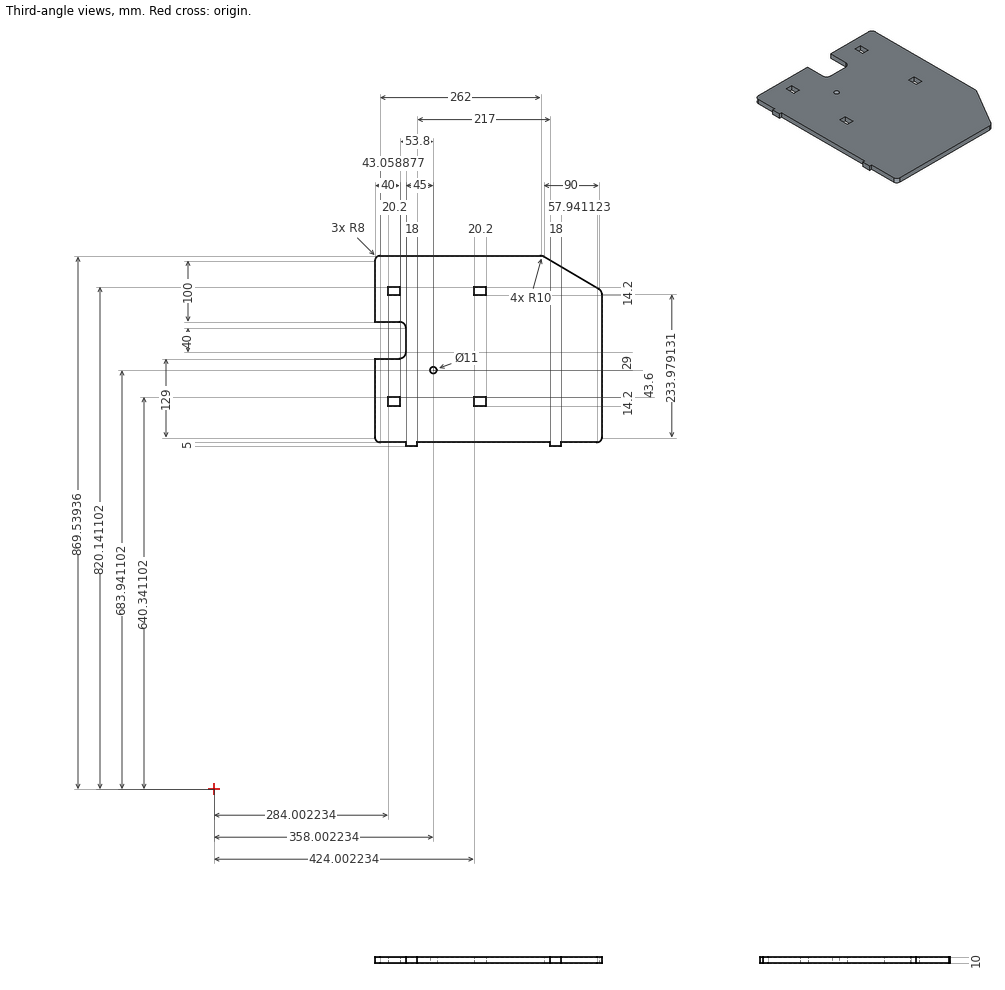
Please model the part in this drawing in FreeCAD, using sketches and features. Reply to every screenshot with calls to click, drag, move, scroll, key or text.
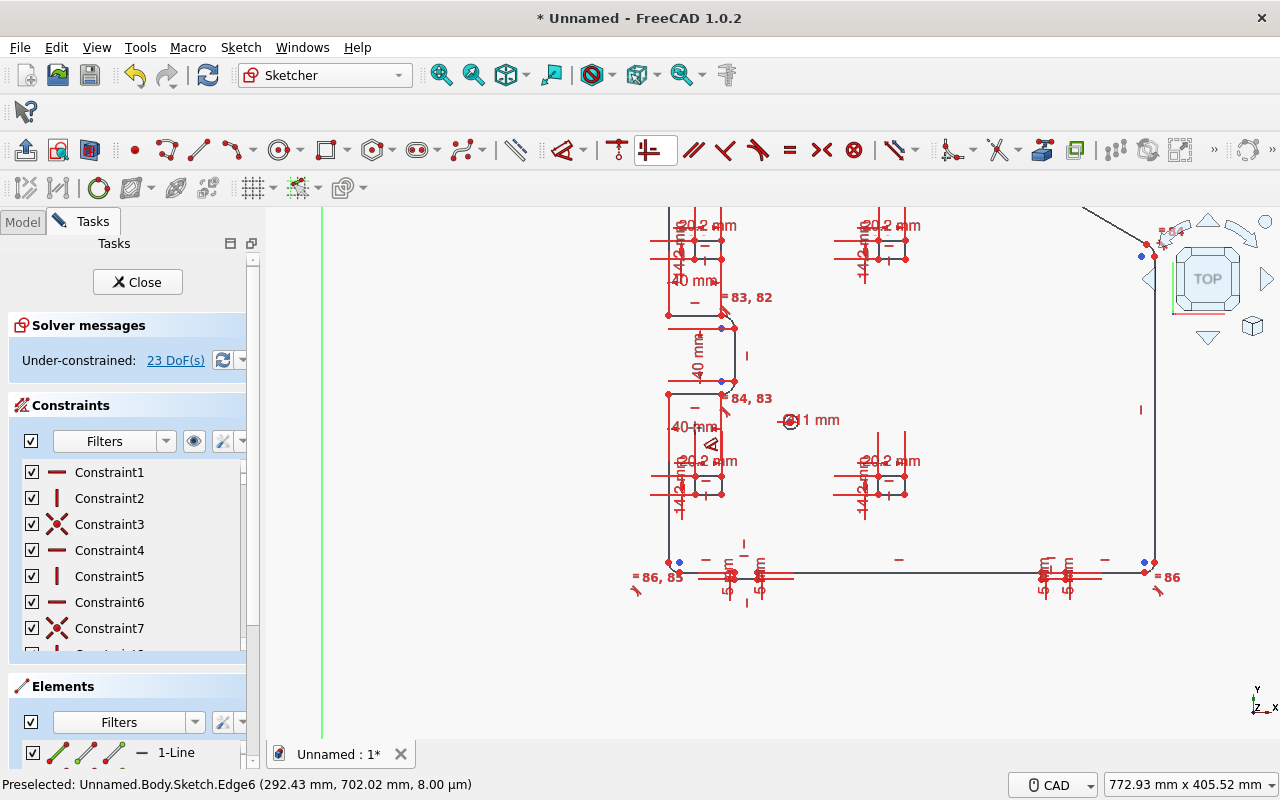
scroll(744, 579, up, 3)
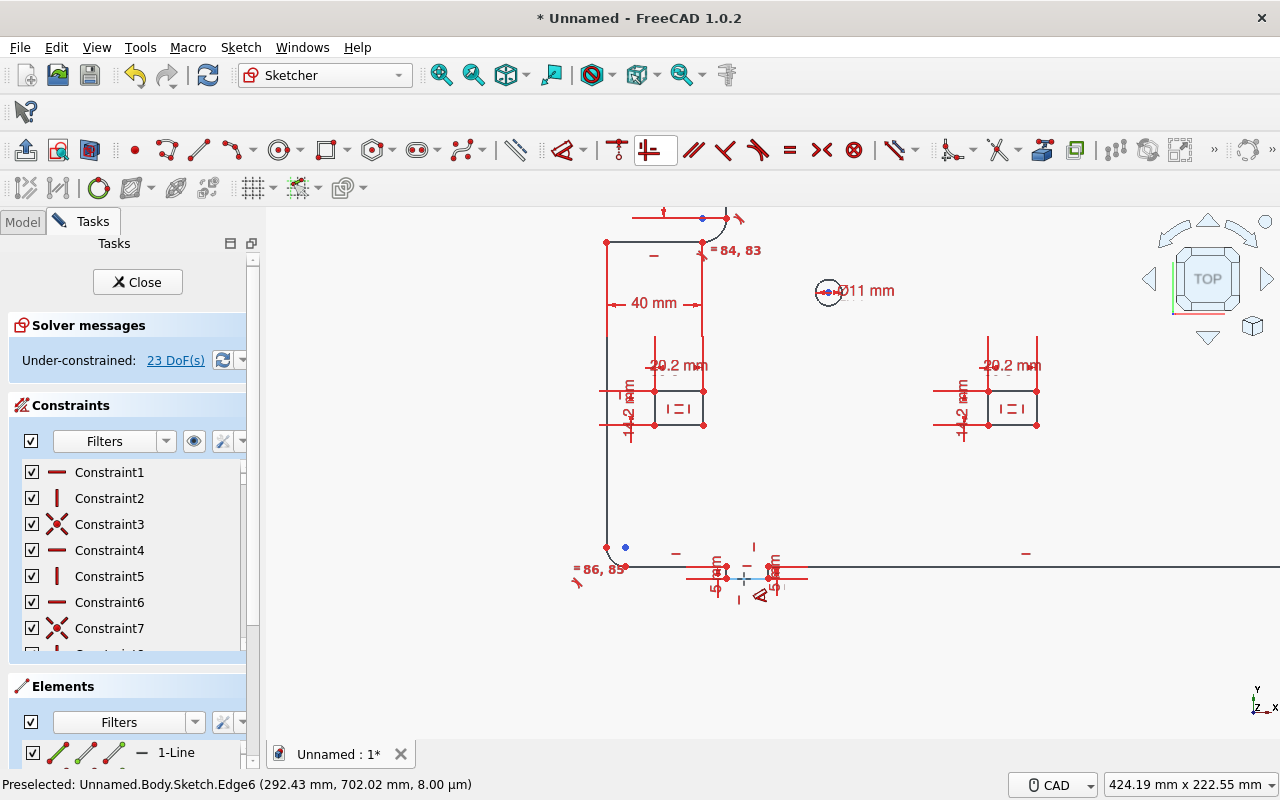
click(743, 579)
click(747, 545)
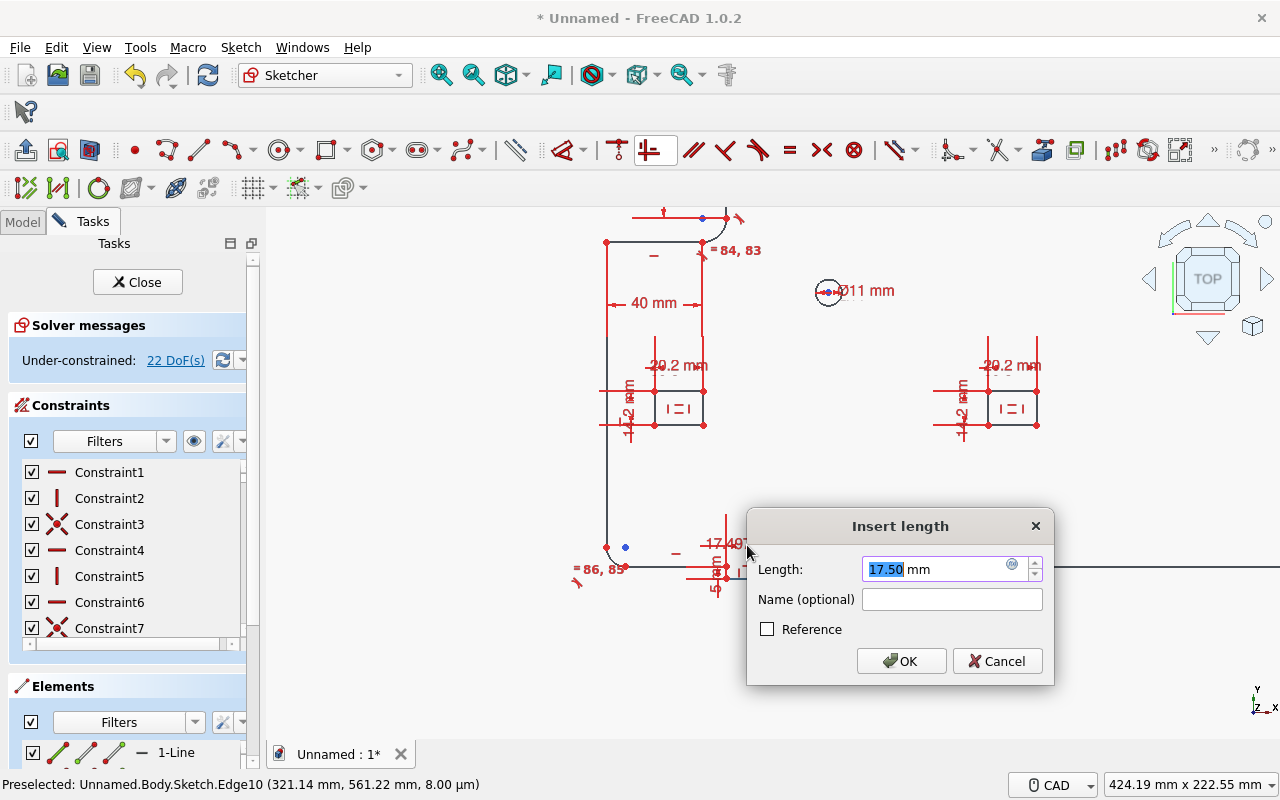
text(18)
key(Return)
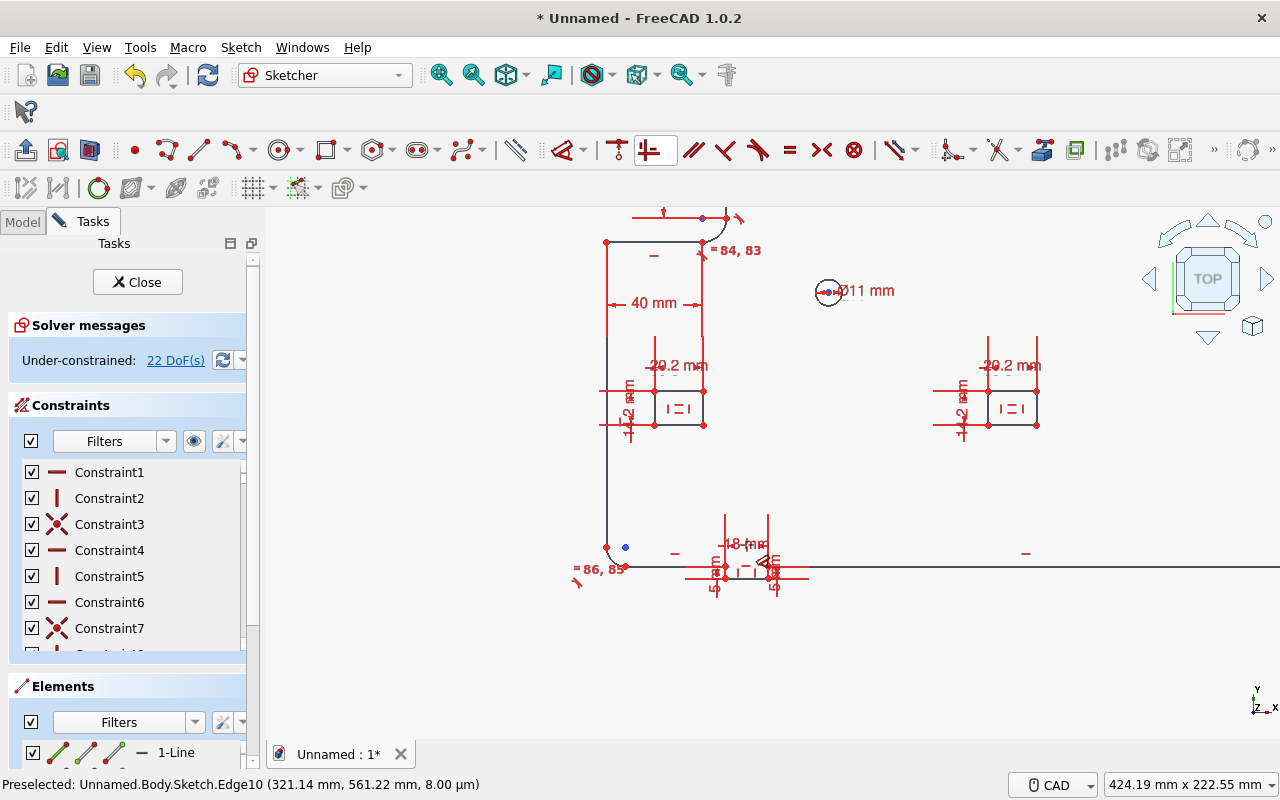
scroll(699, 393, down, 9)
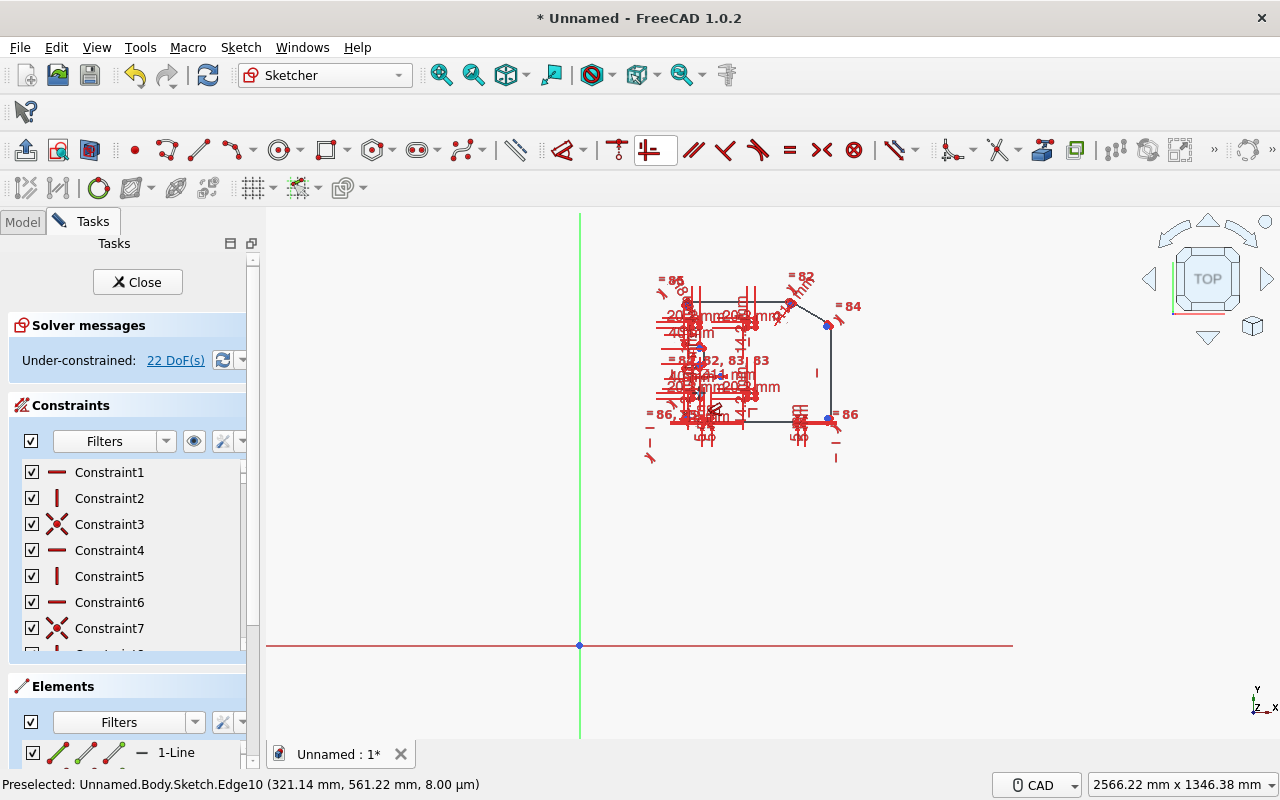
scroll(798, 424, up, 10)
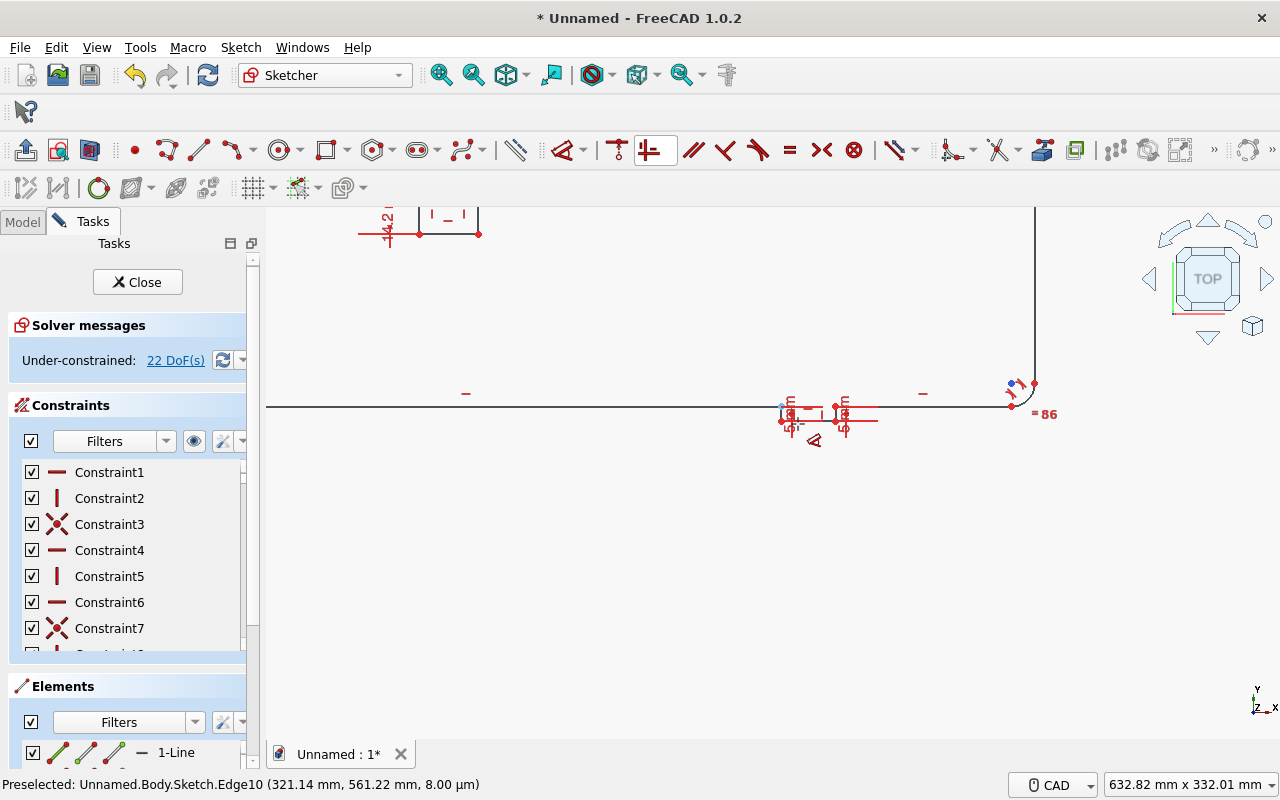
click(798, 421)
click(809, 387)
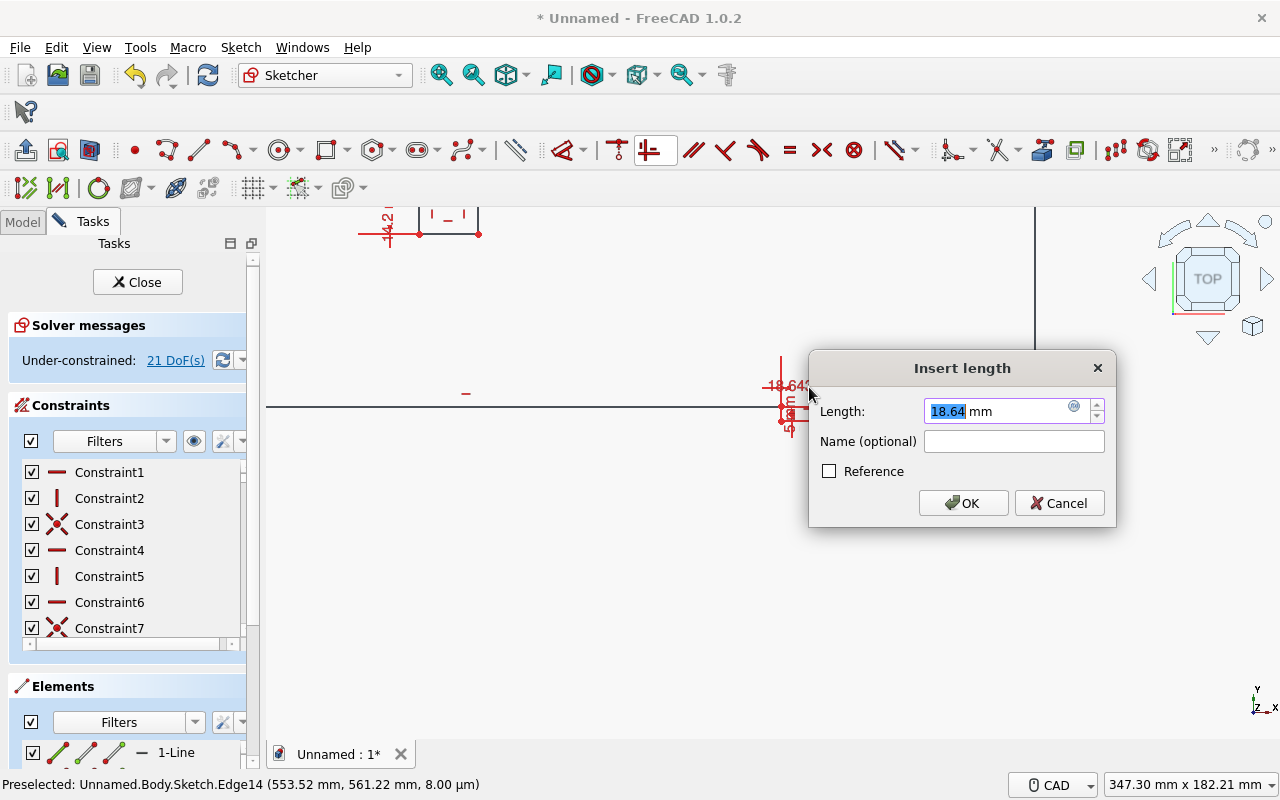
text(18)
key(Return)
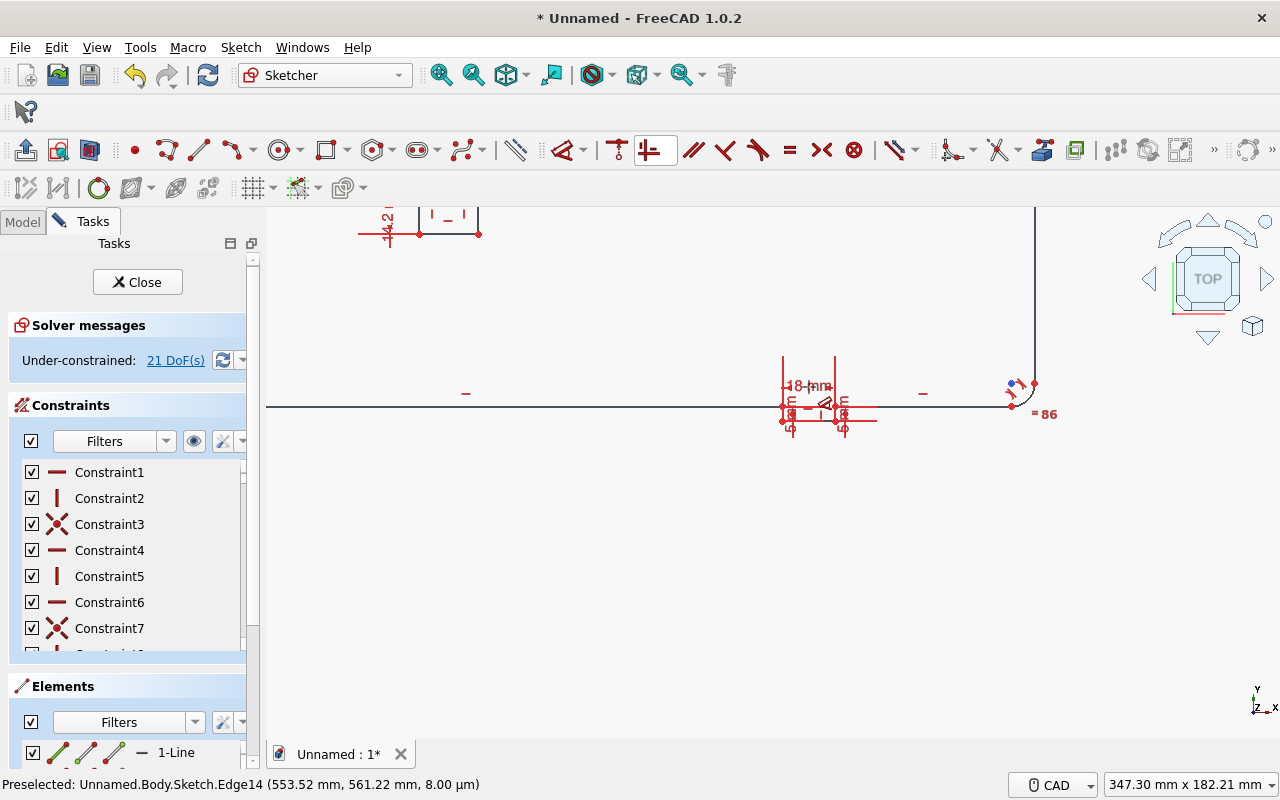
scroll(798, 424, down, 10)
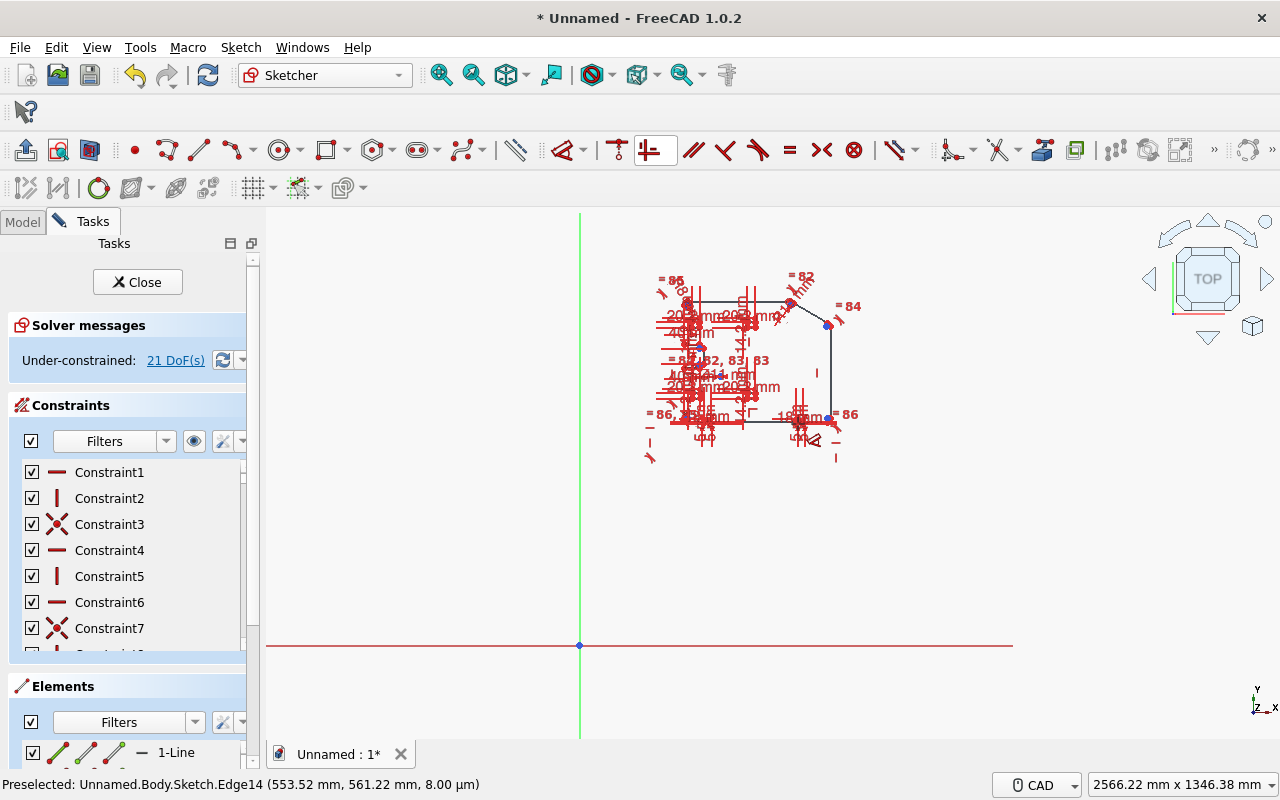
click(760, 302)
click(739, 268)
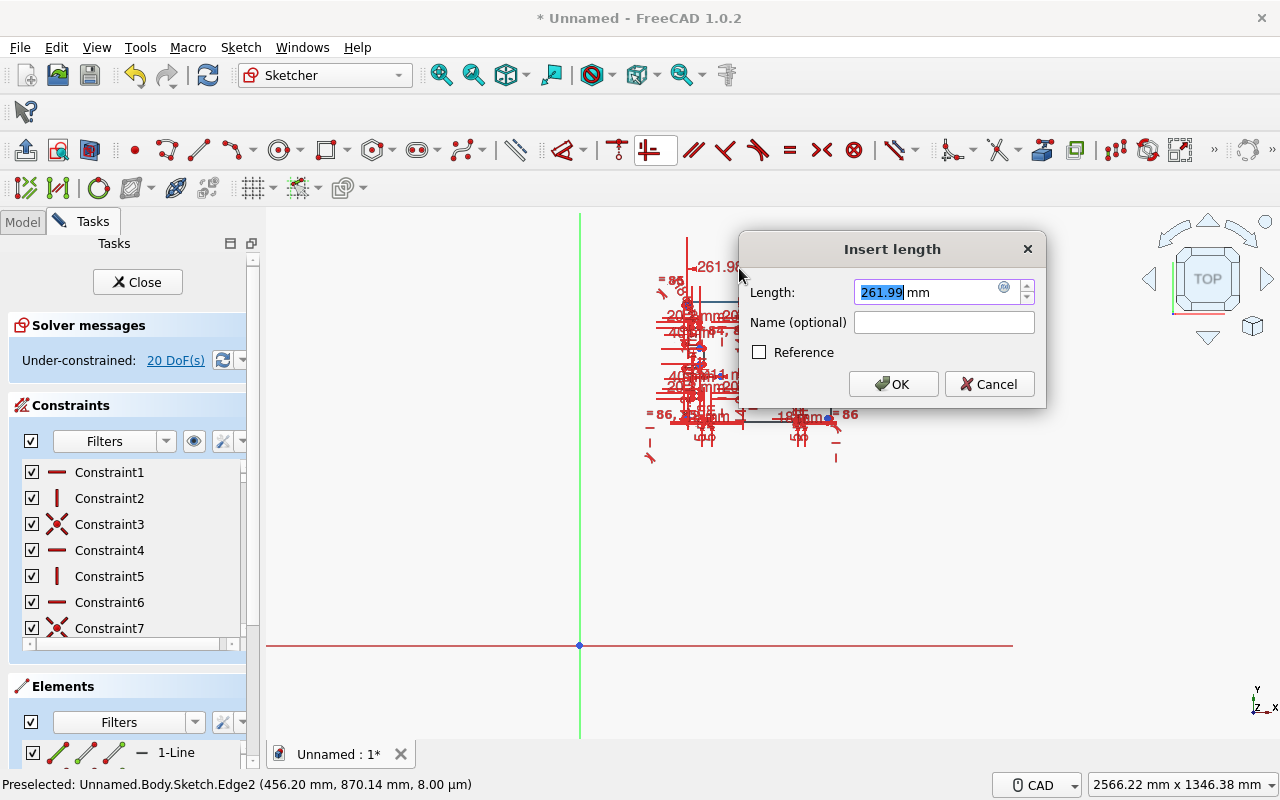
text(262)
key(Return)